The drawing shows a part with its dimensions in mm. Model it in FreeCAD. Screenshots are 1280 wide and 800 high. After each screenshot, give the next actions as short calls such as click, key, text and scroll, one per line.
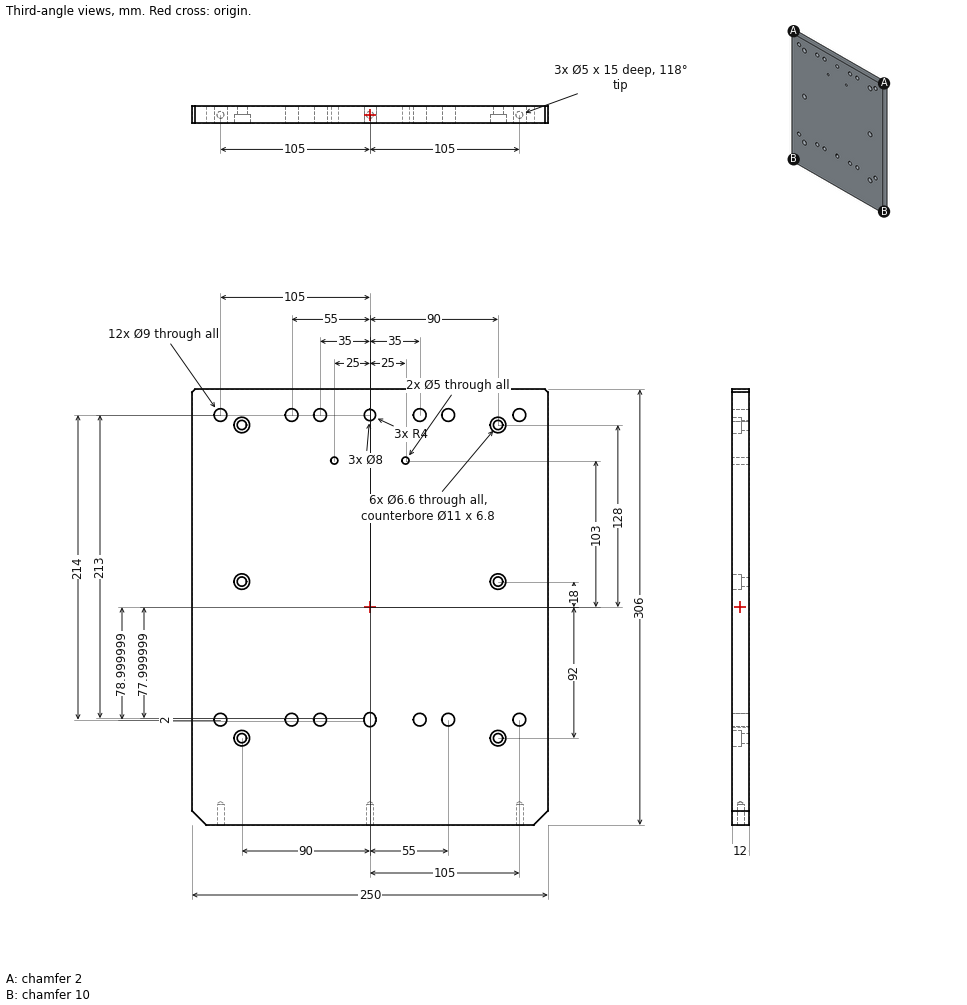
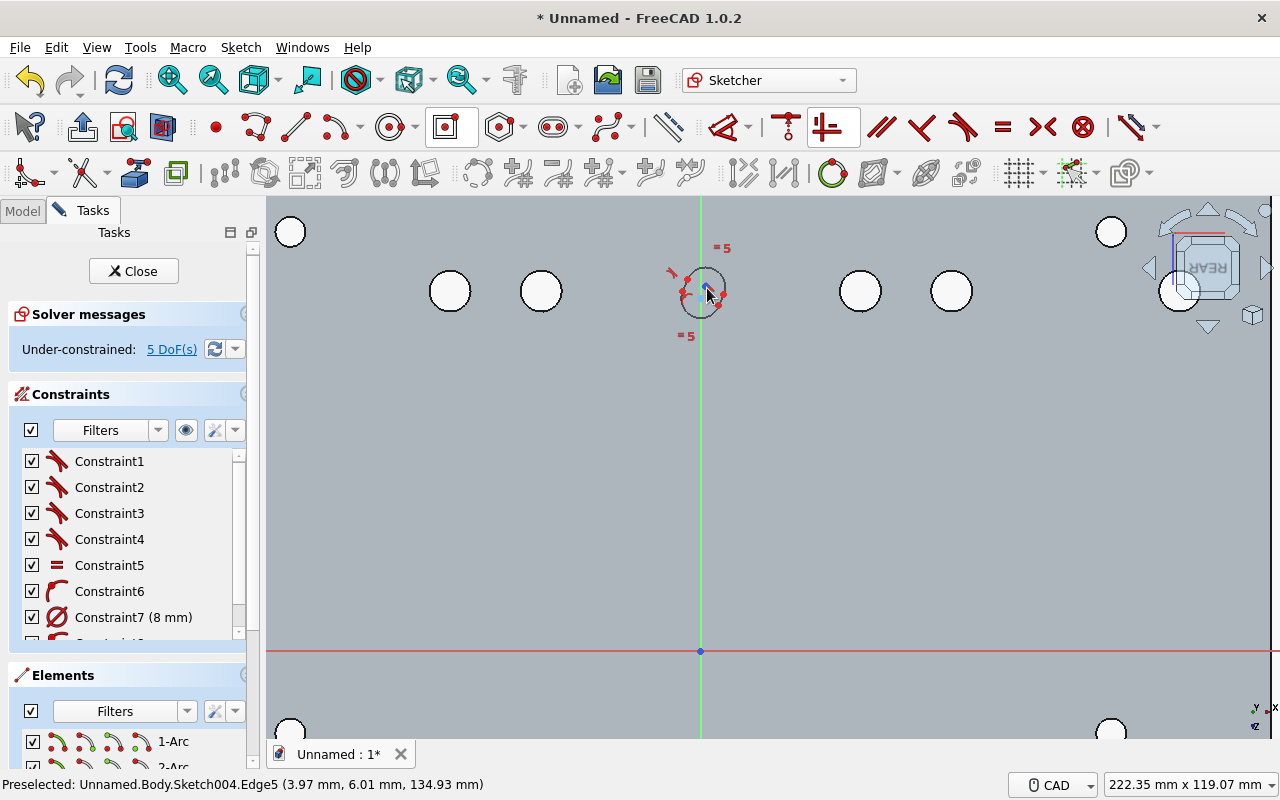
click(706, 287)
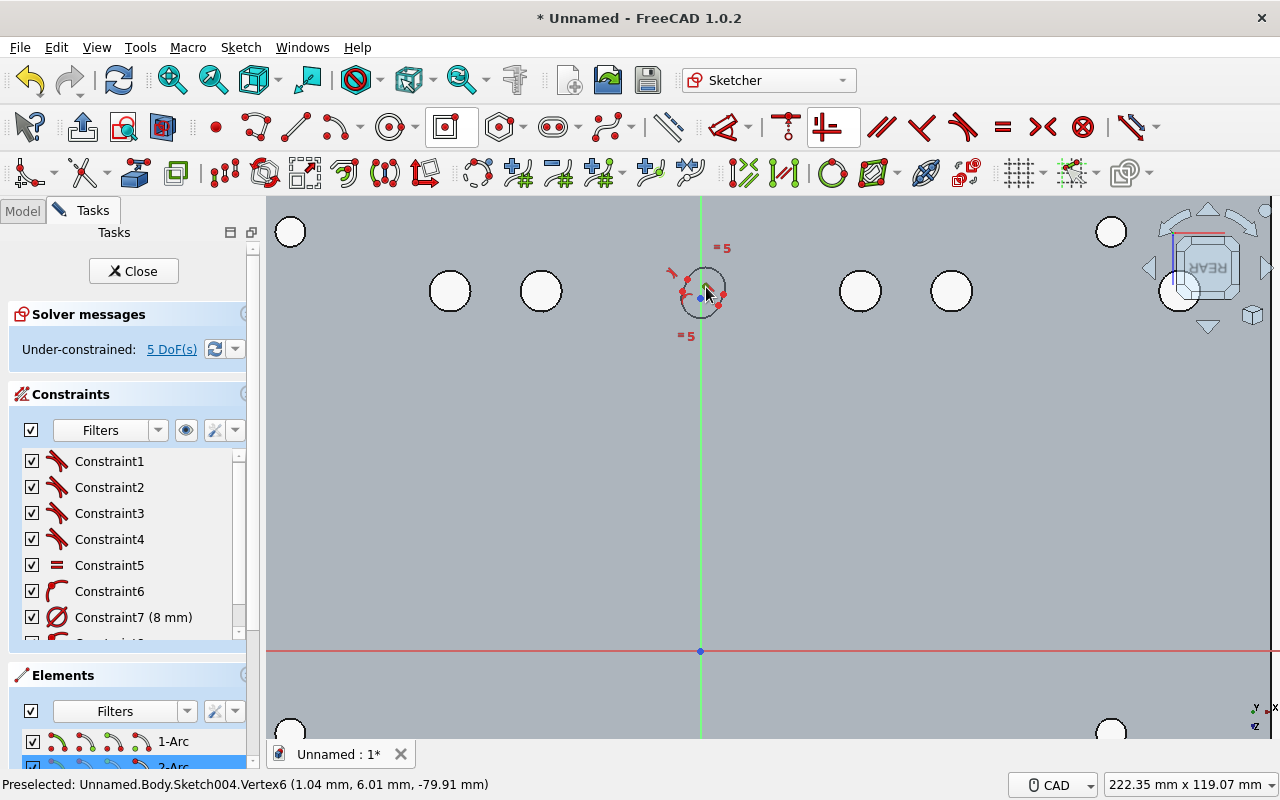
click(701, 607)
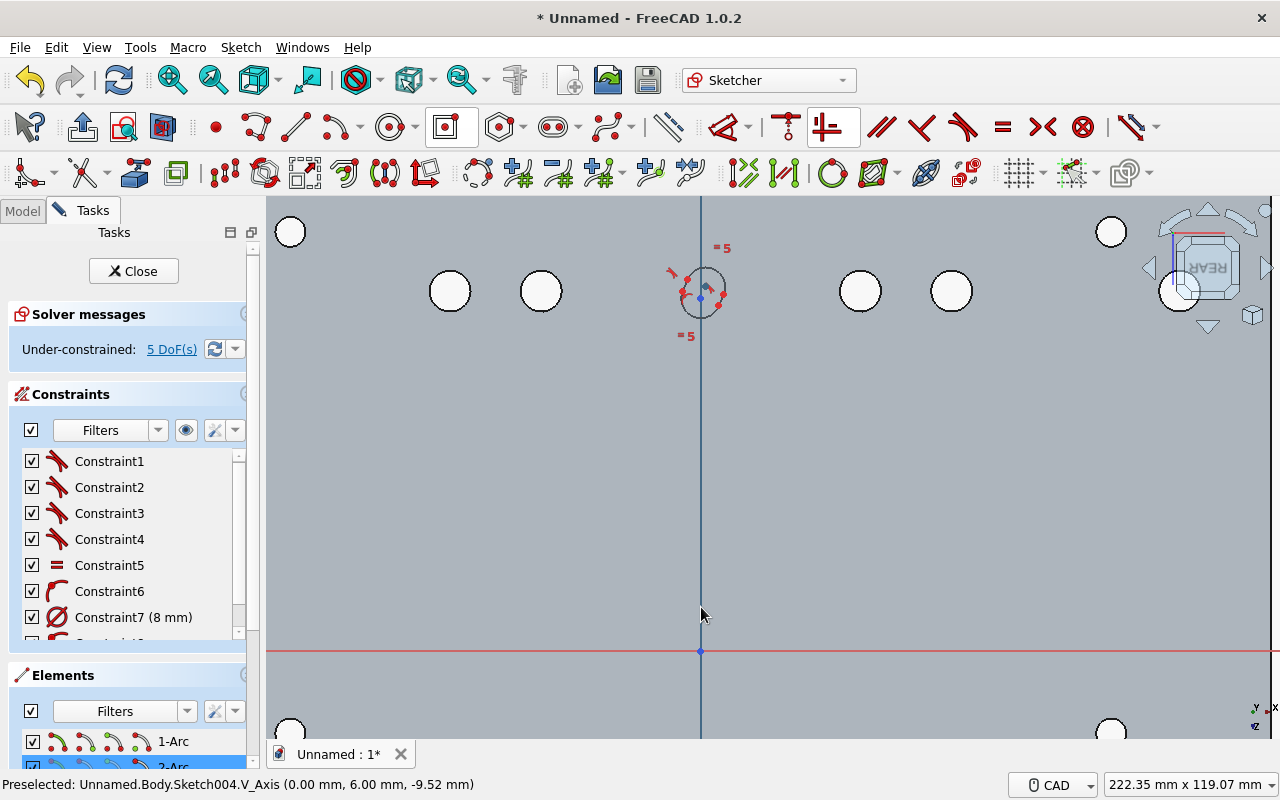
key(c)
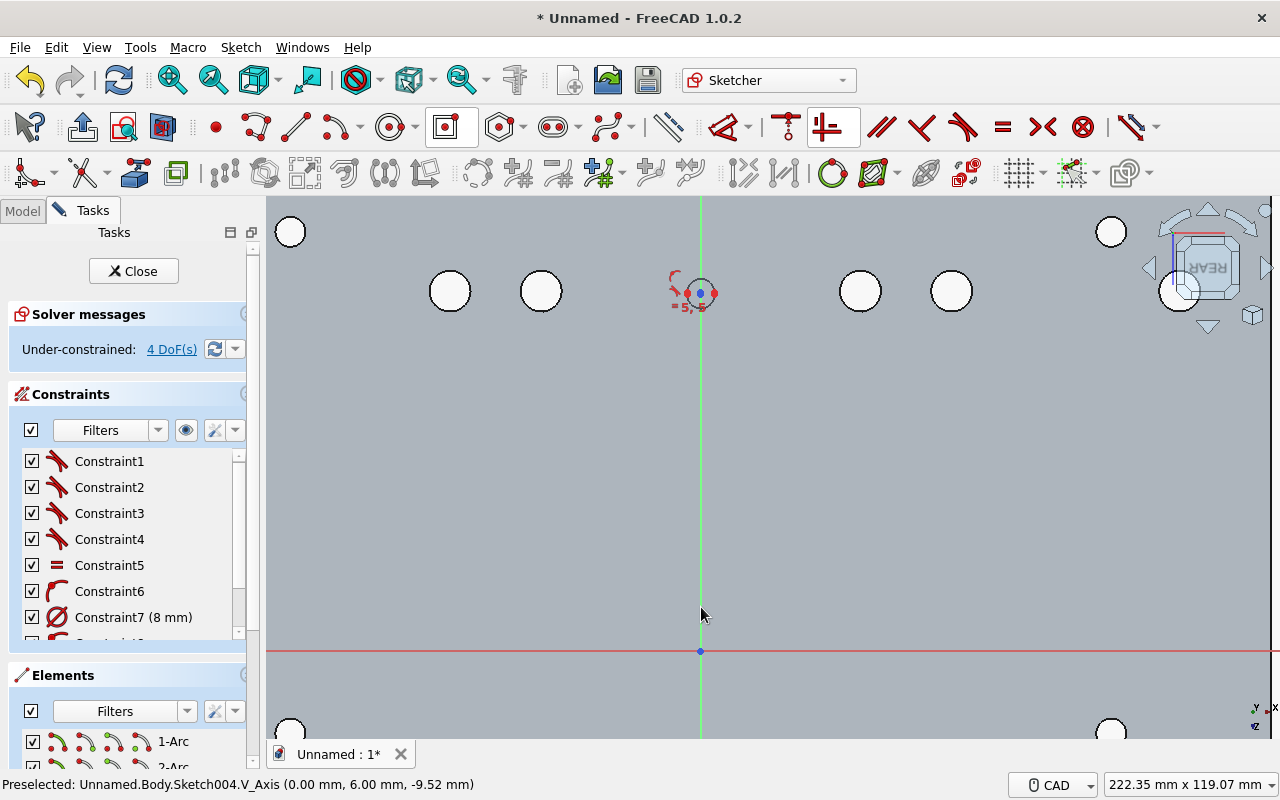
click(724, 128)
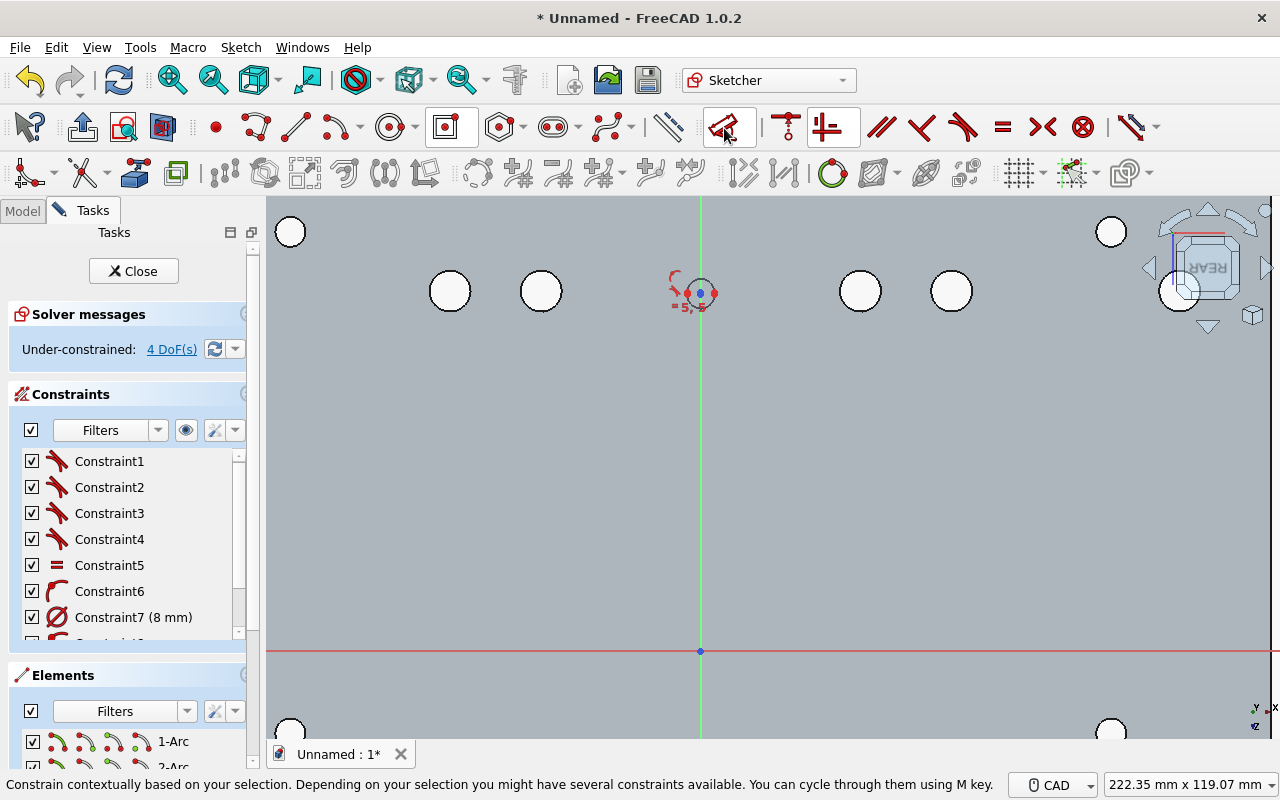
scroll(701, 309, up, 4)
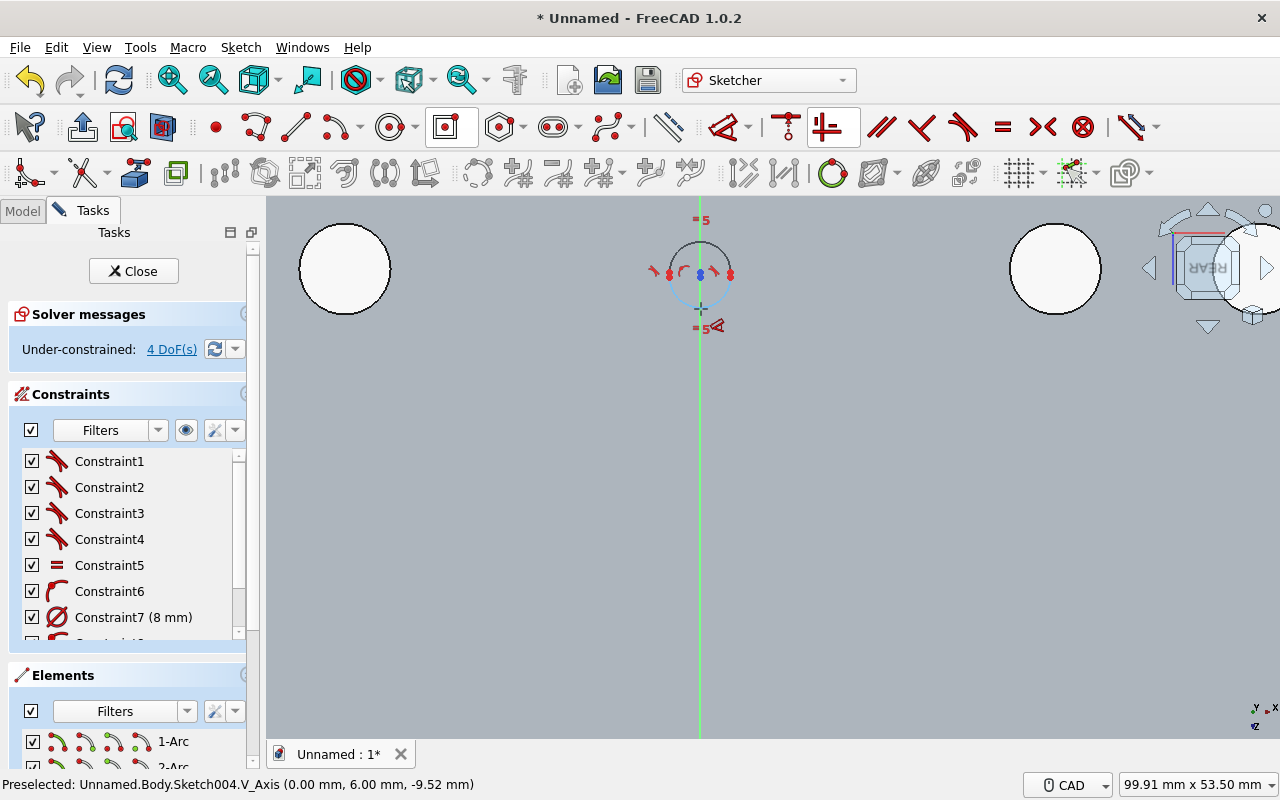
click(700, 308)
click(670, 332)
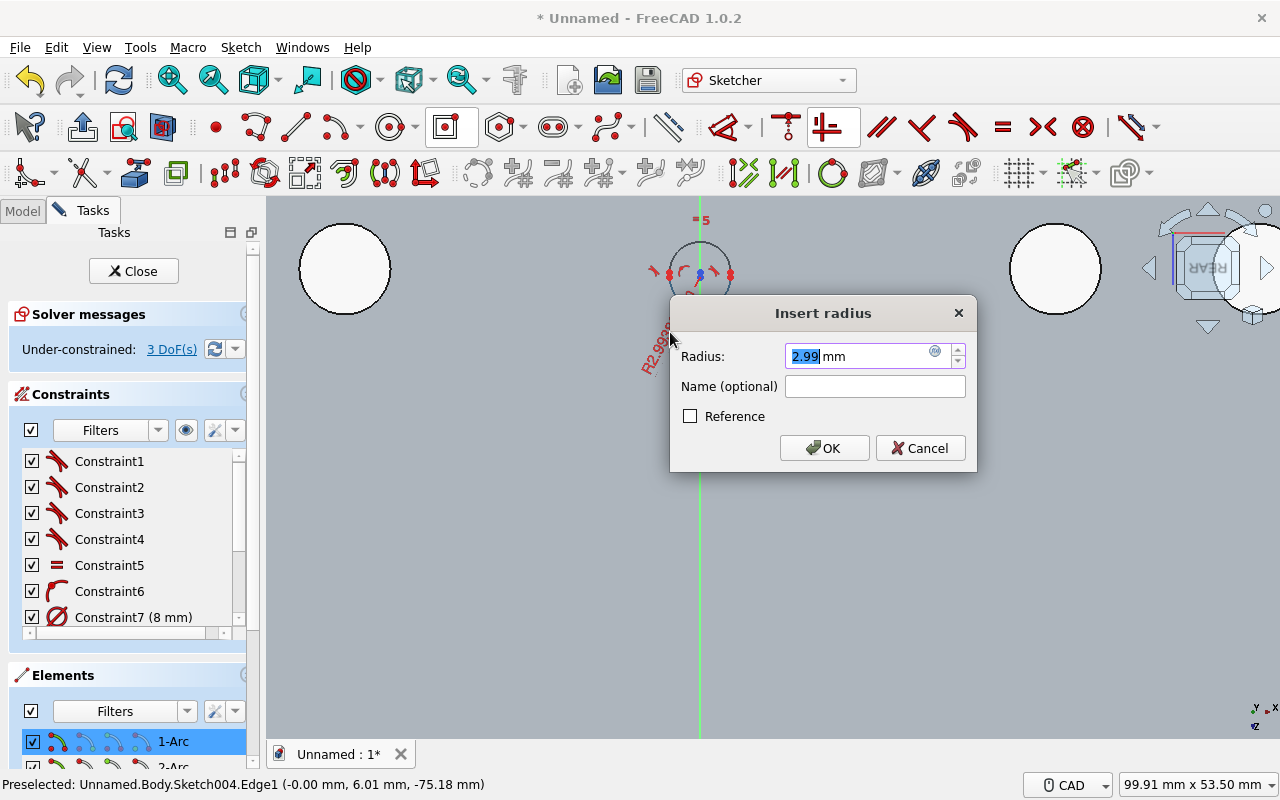
text(4)
key(Return)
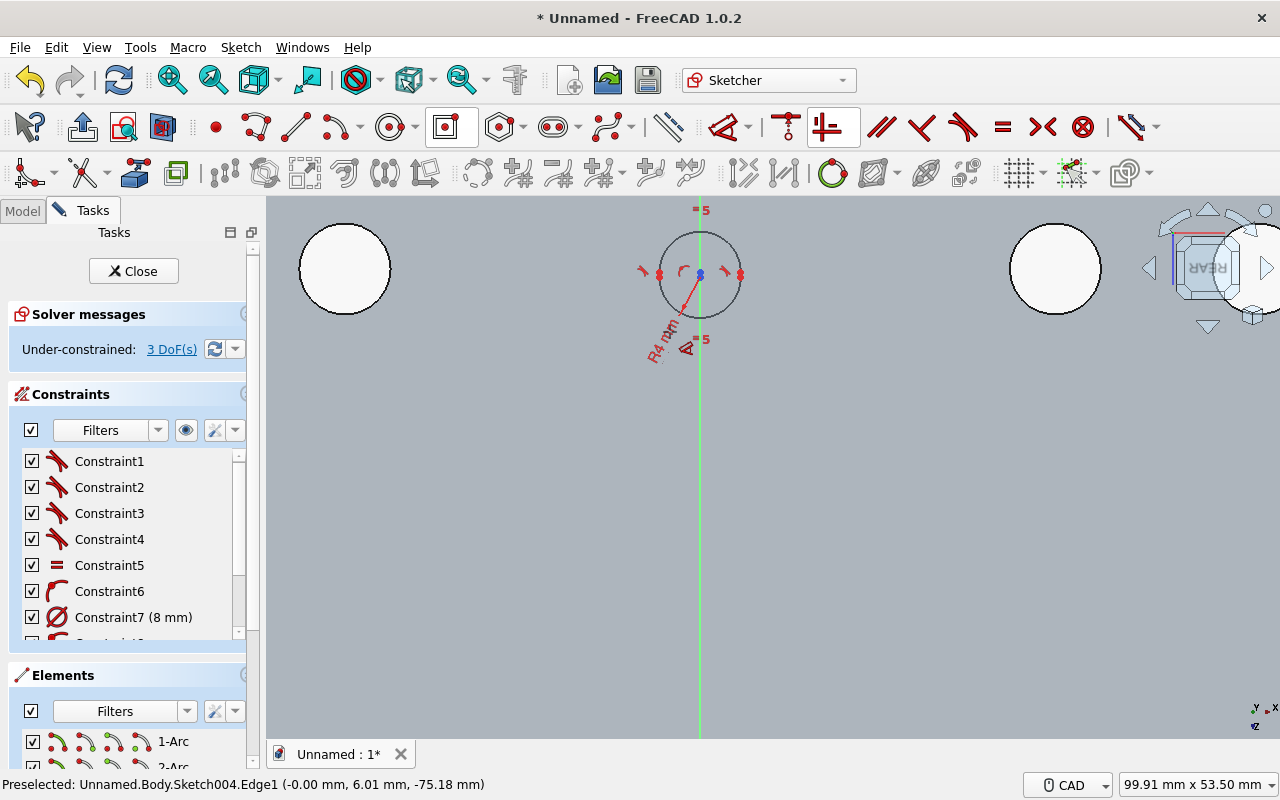
scroll(660, 275, up, 4)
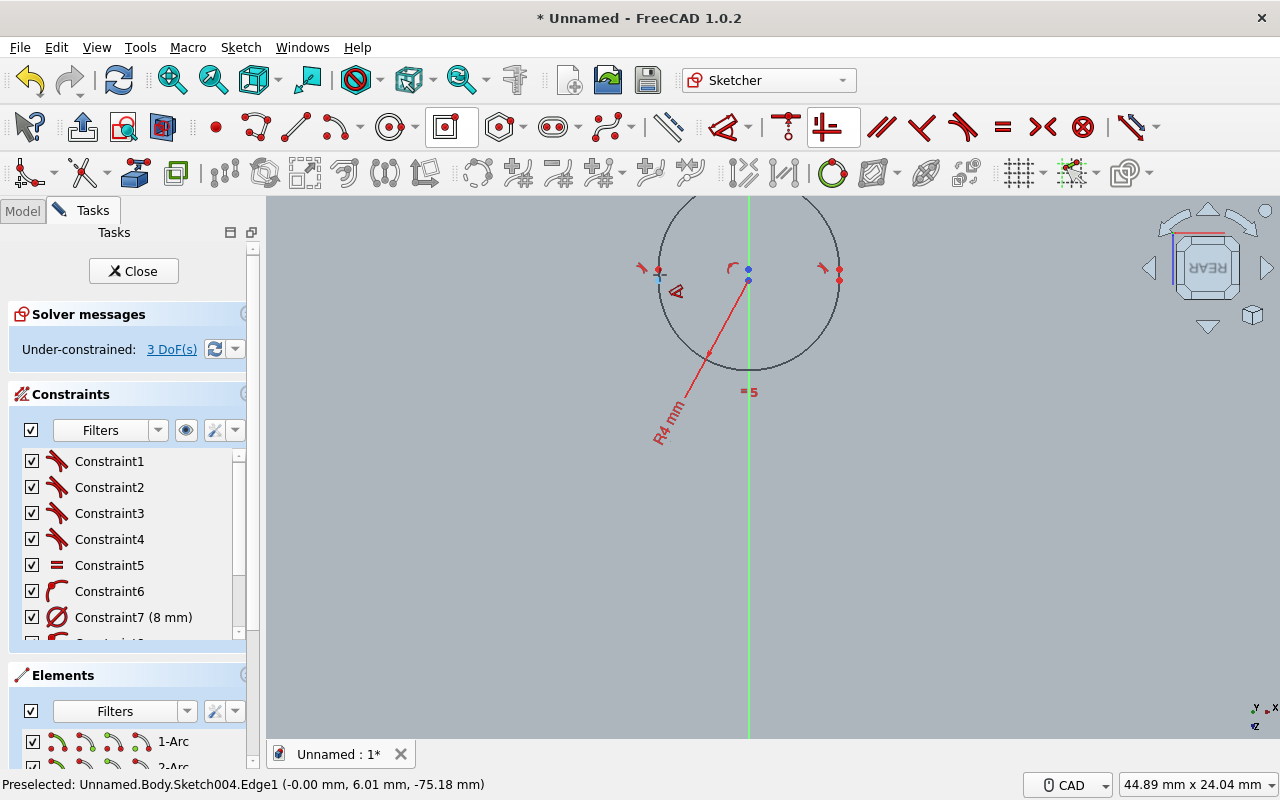
click(659, 273)
click(625, 275)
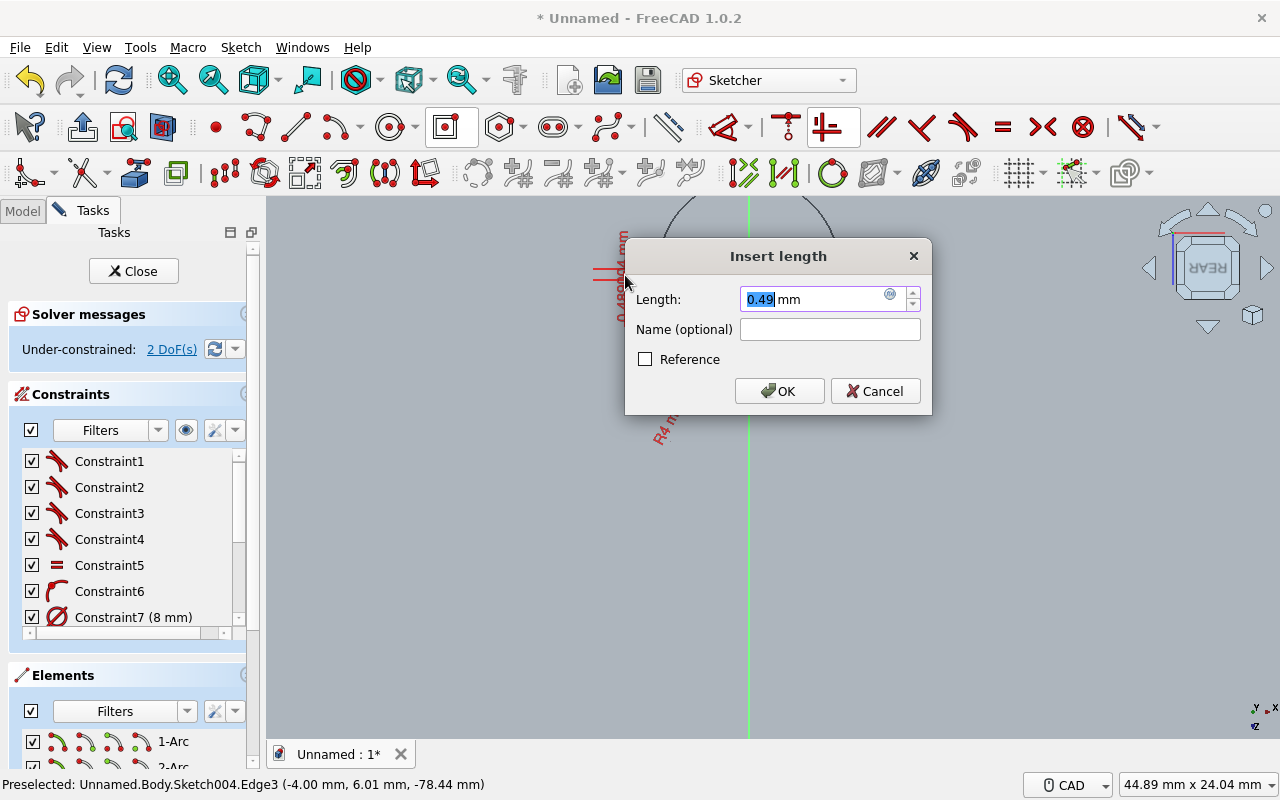
text(2)
key(Return)